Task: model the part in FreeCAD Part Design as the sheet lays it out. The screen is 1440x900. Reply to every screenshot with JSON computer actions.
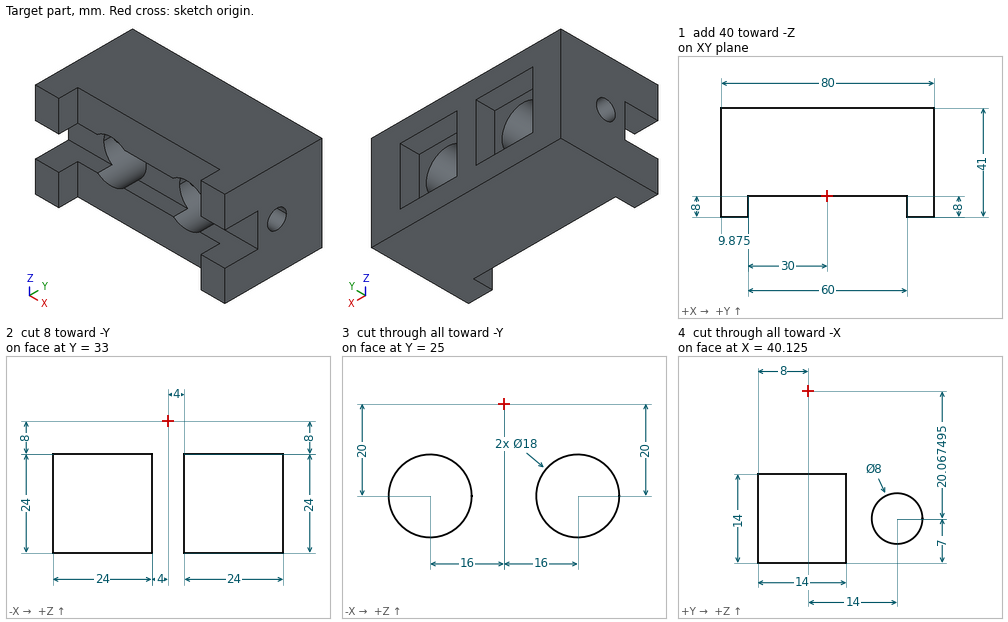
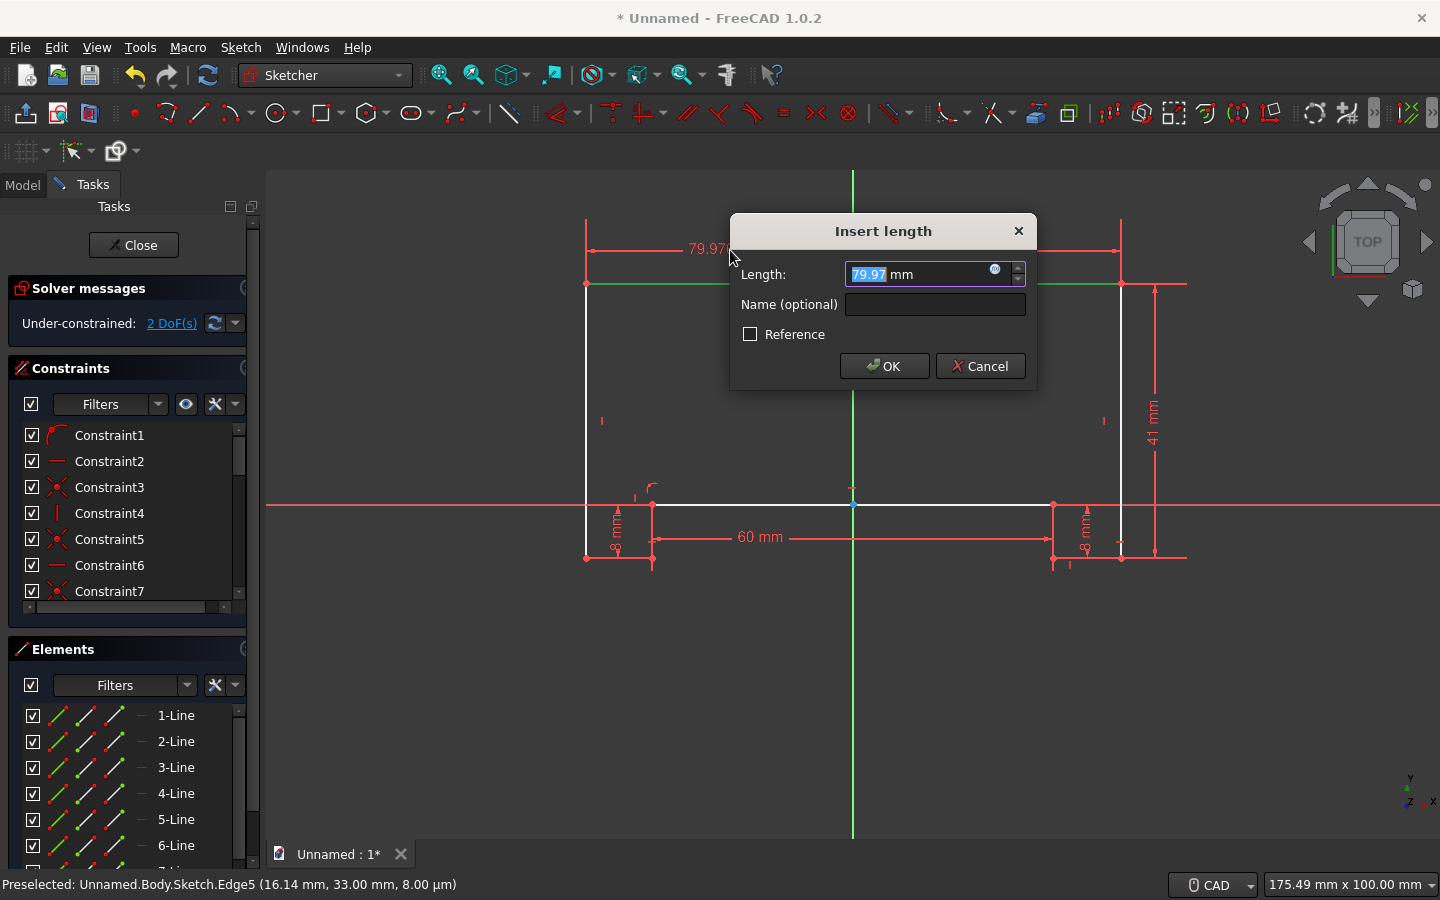
{"action": "type", "text": "80"}
{"action": "key", "text": "Return"}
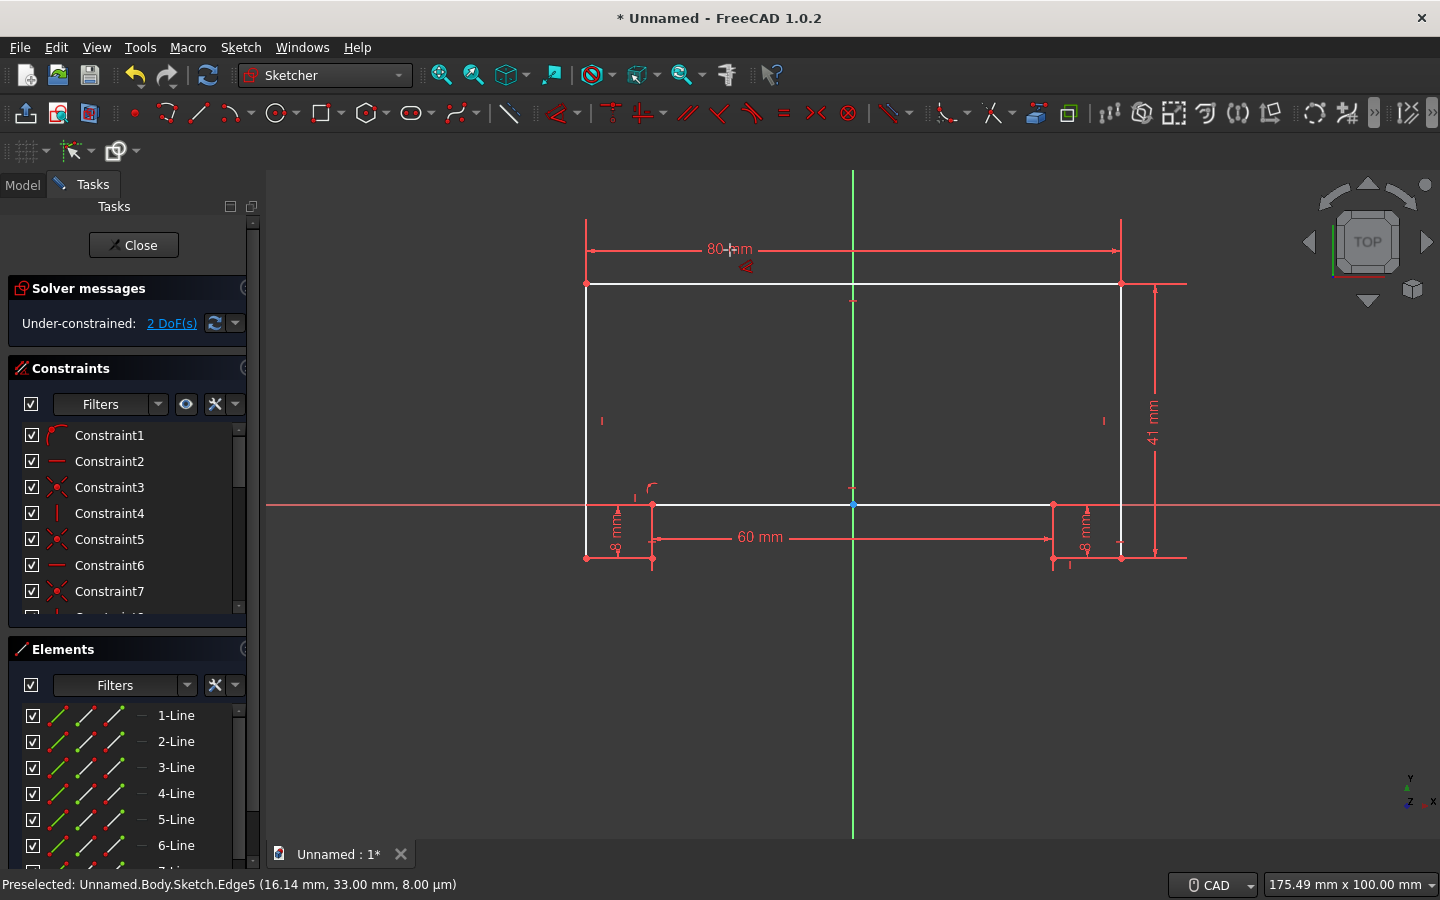
{"action": "left_click", "coordinate": [652, 504]}
{"action": "left_click", "coordinate": [752, 470]}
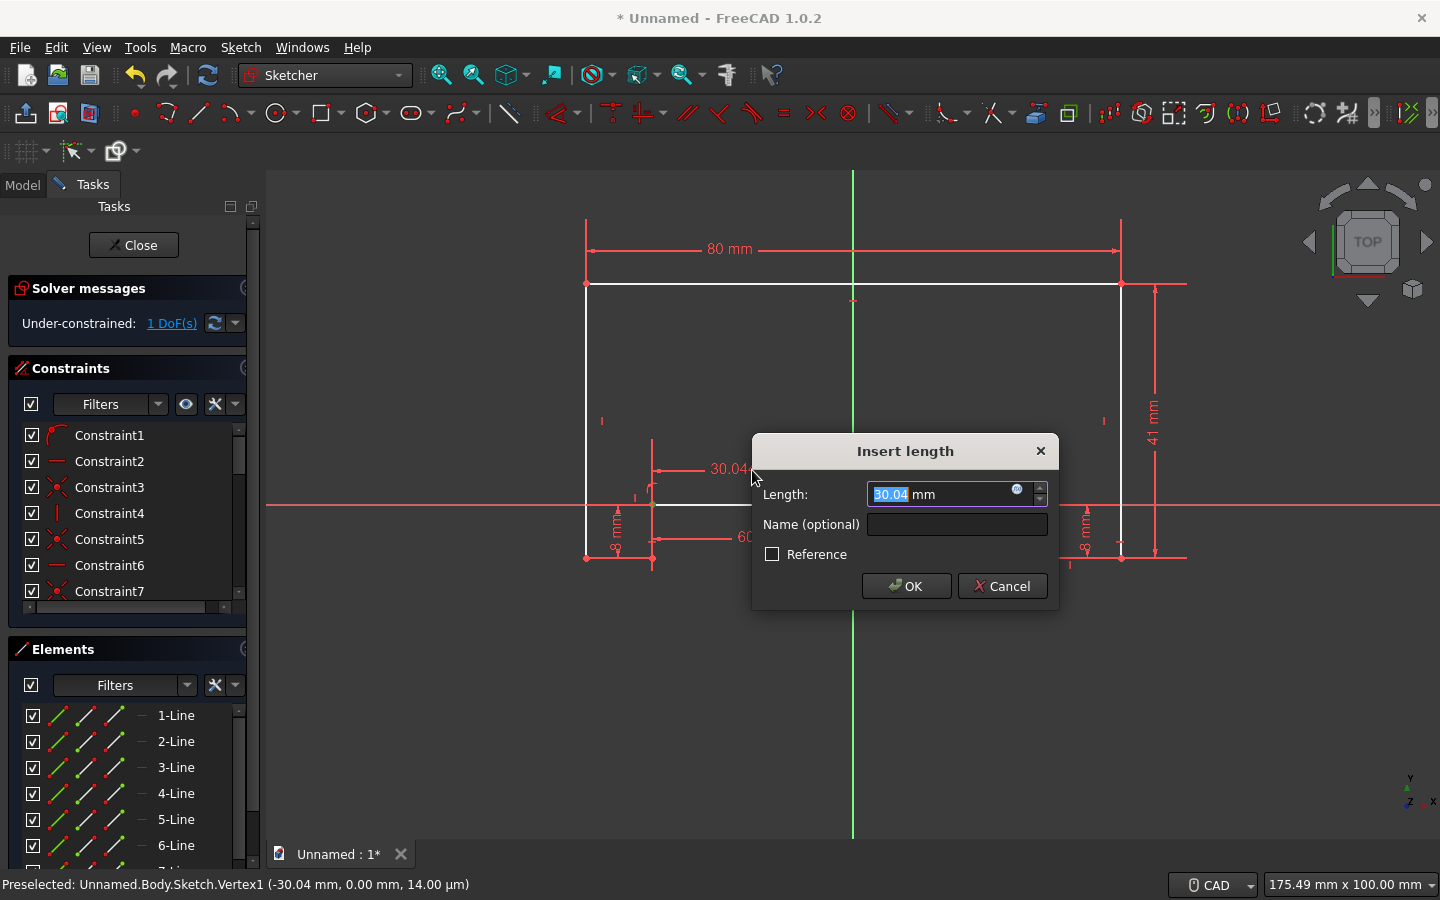
{"action": "type", "text": "30"}
{"action": "key", "text": "Return"}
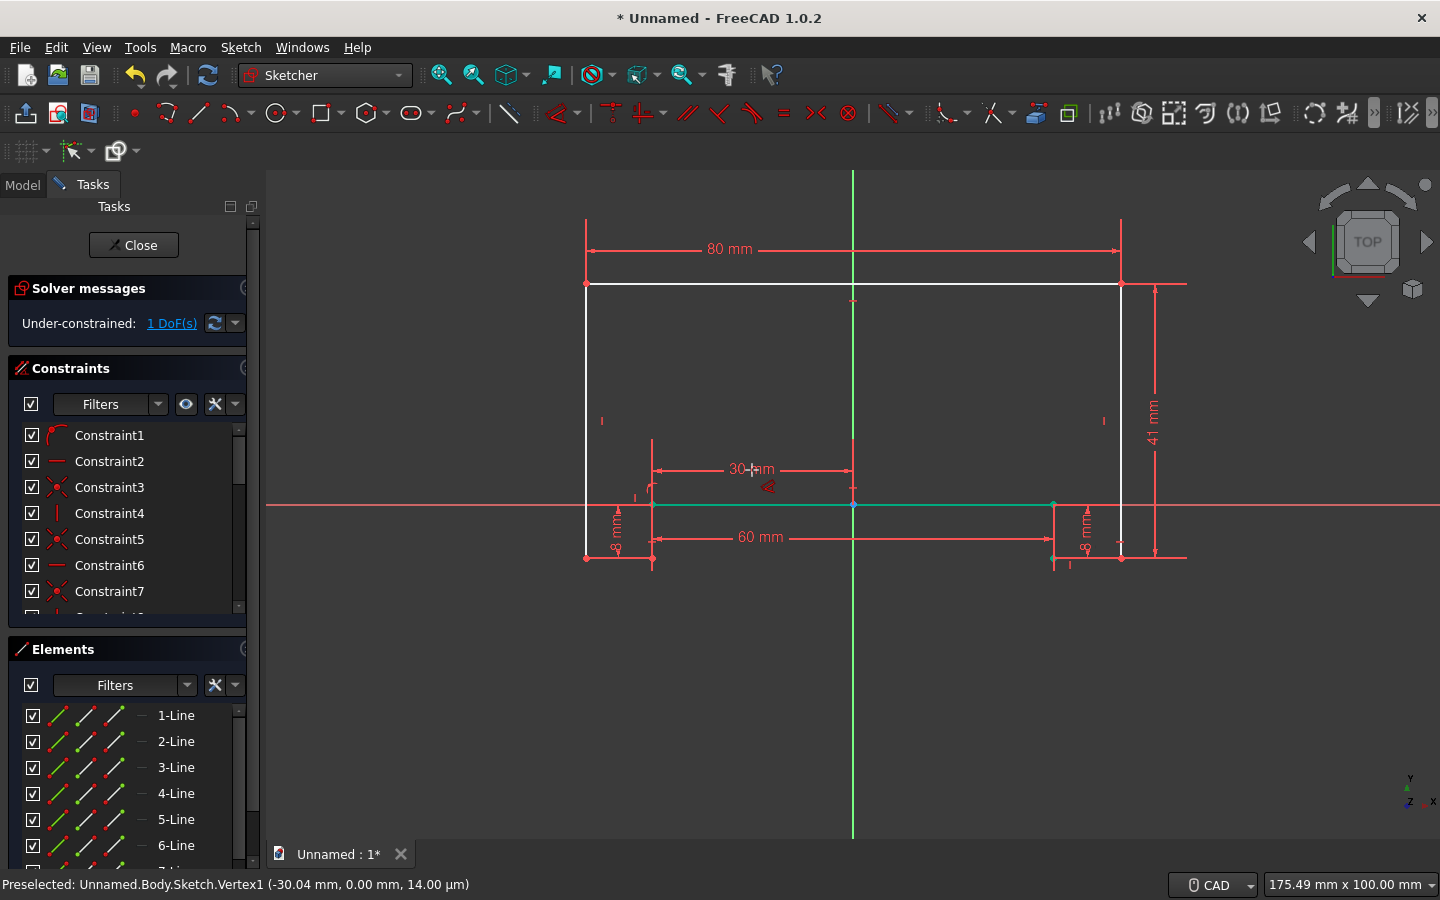
{"action": "left_click", "coordinate": [606, 558]}
{"action": "left_click", "coordinate": [619, 592]}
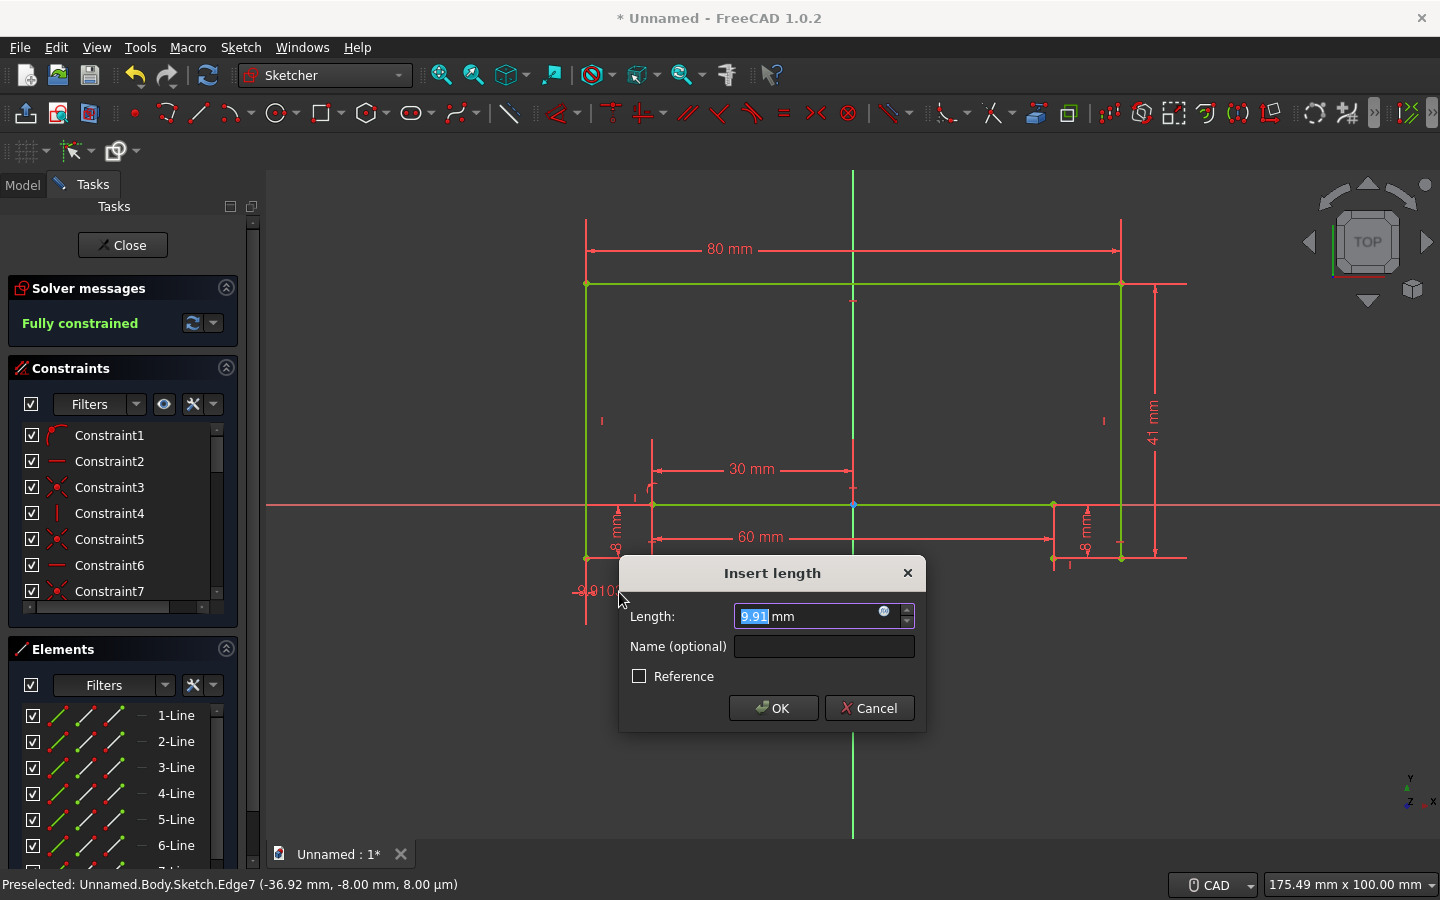
{"action": "type", "text": "9.875"}
{"action": "key", "text": "Return"}
{"action": "key", "text": "Escape"}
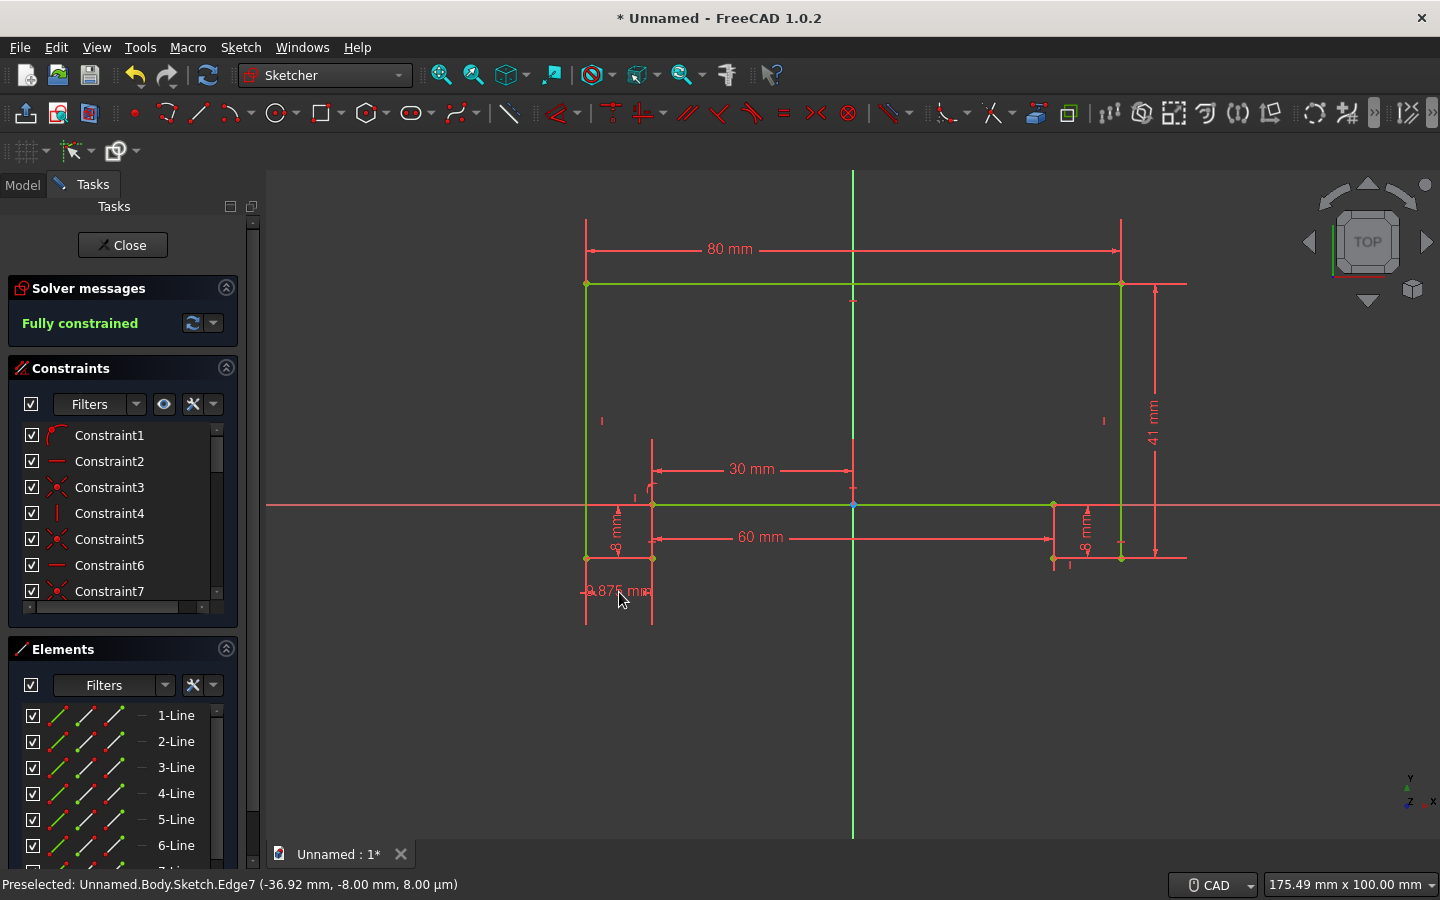
{"action": "left_click", "coordinate": [123, 245]}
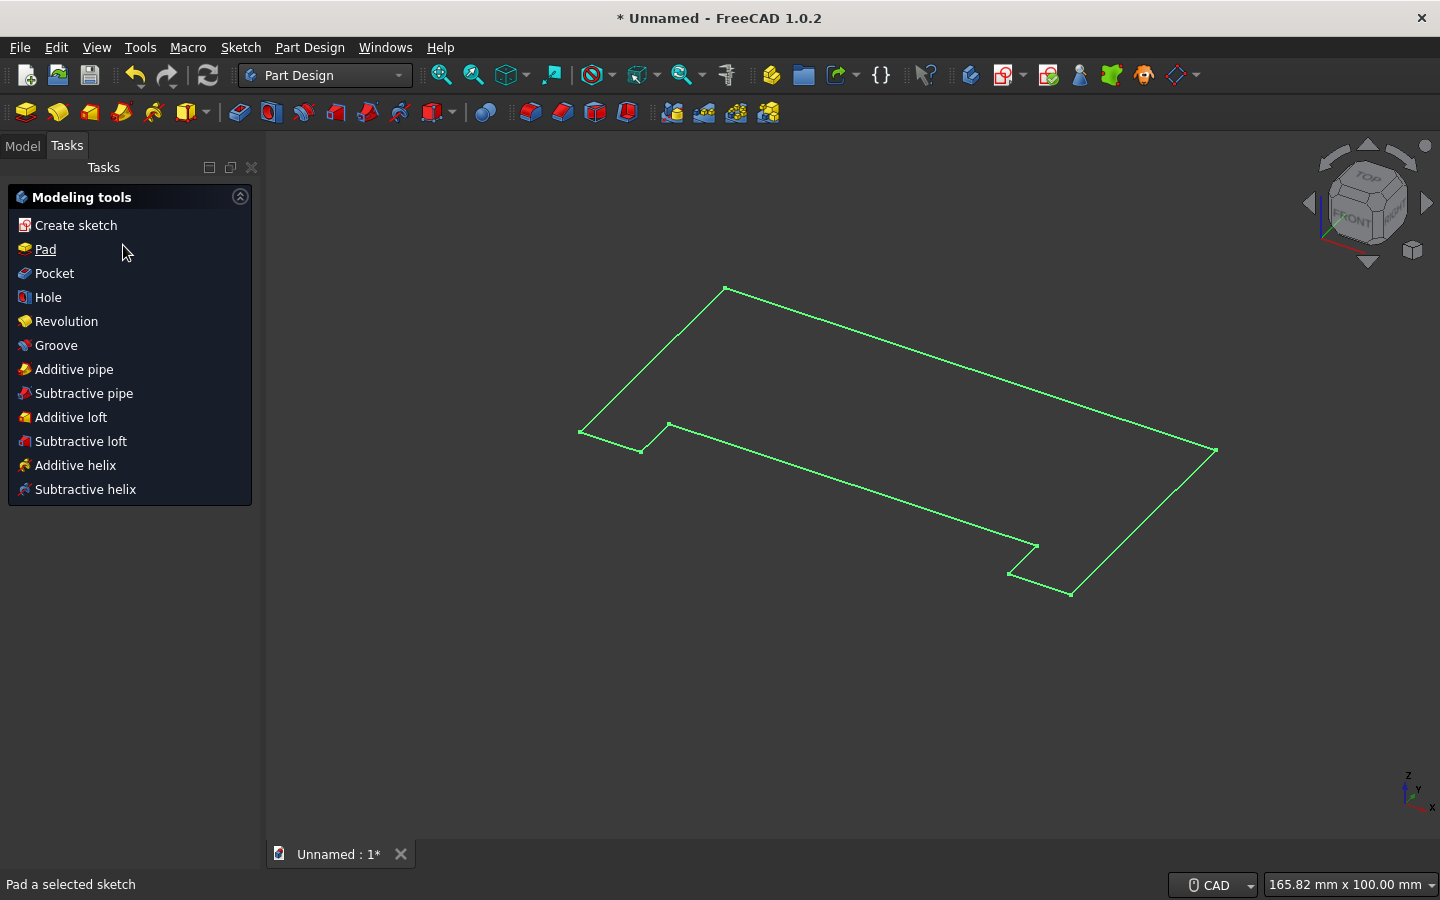
{"action": "left_click", "coordinate": [26, 112]}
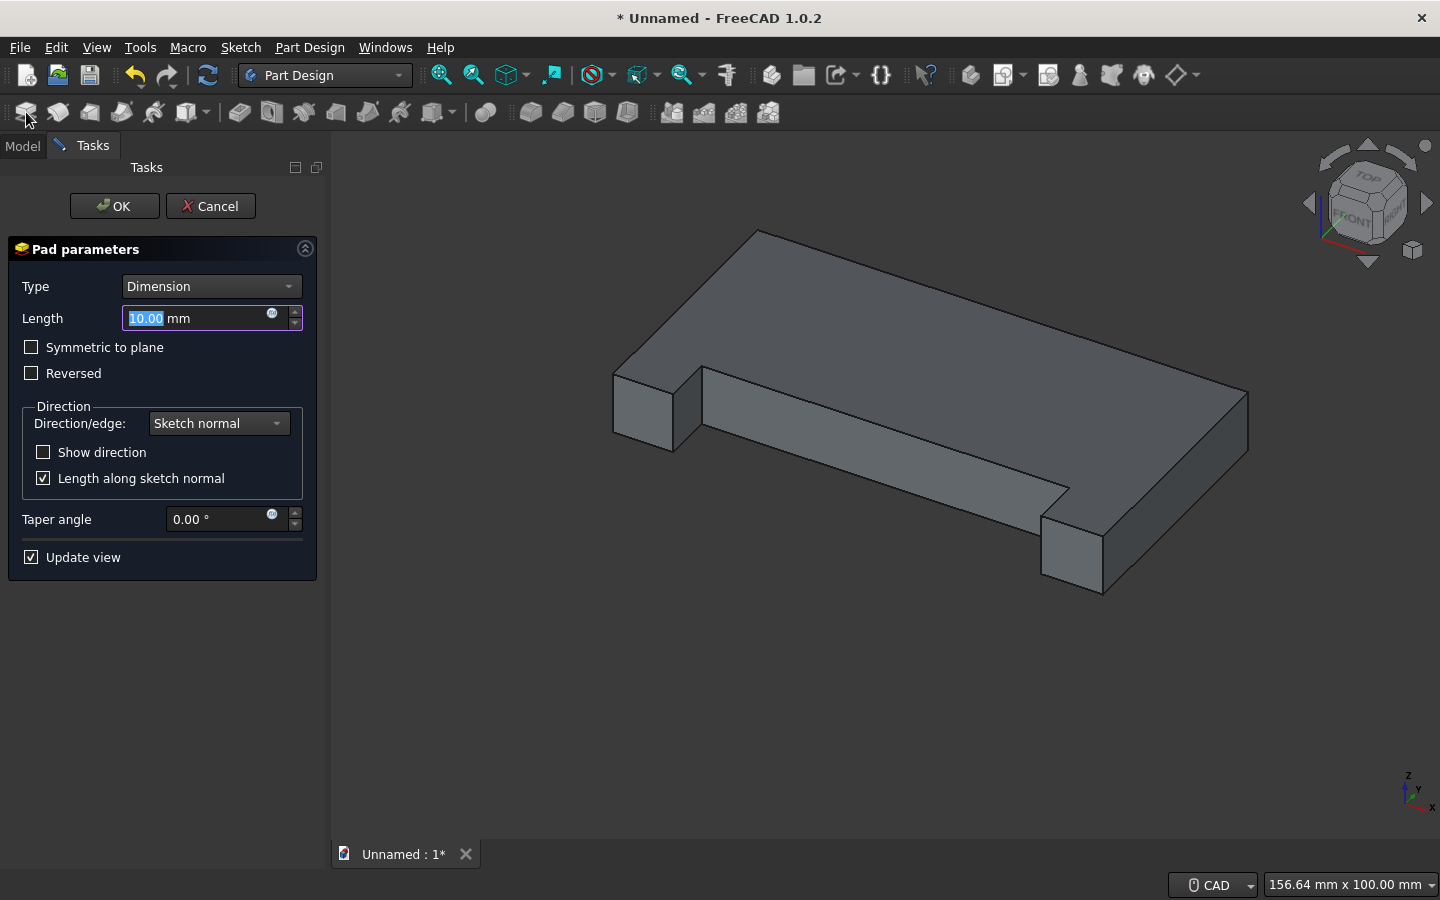
{"action": "type", "text": "40"}
{"action": "key", "text": "Tab"}